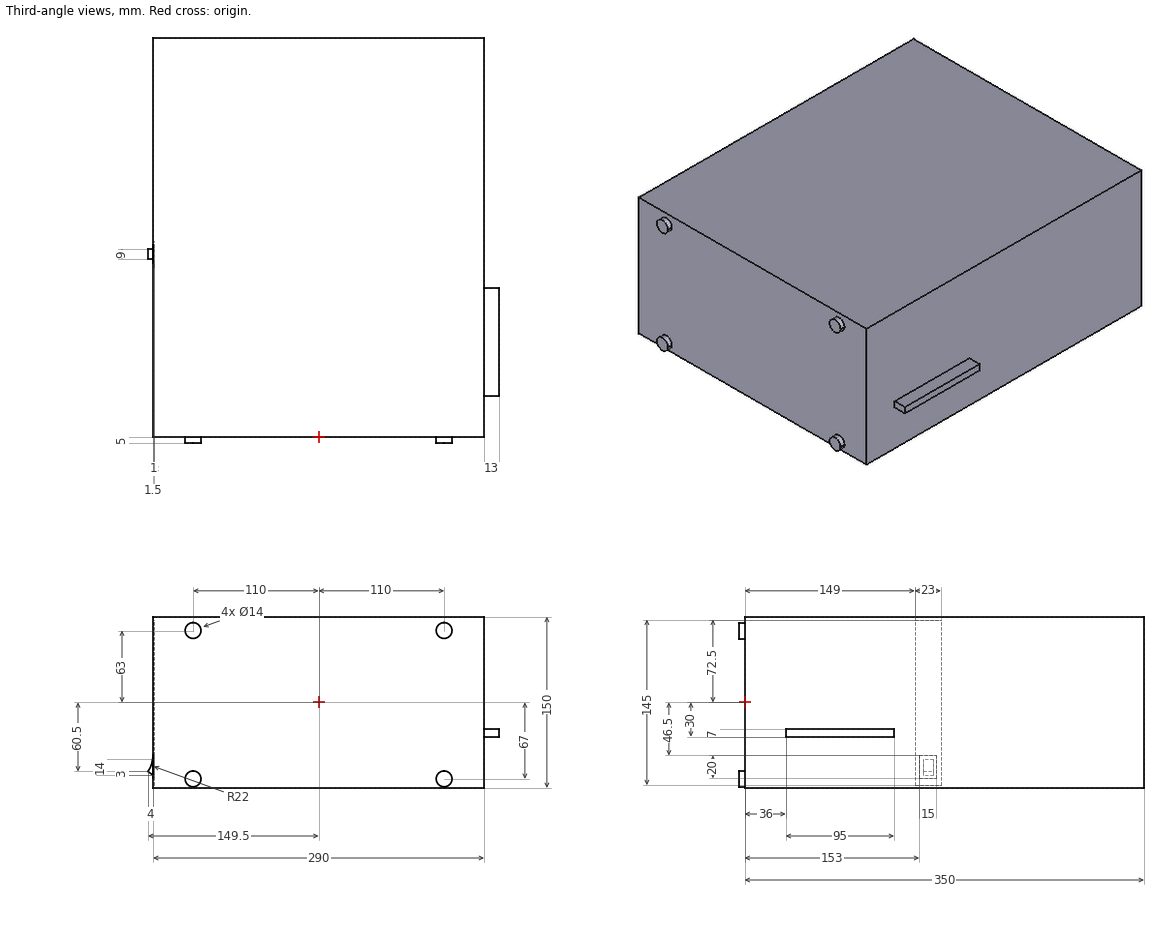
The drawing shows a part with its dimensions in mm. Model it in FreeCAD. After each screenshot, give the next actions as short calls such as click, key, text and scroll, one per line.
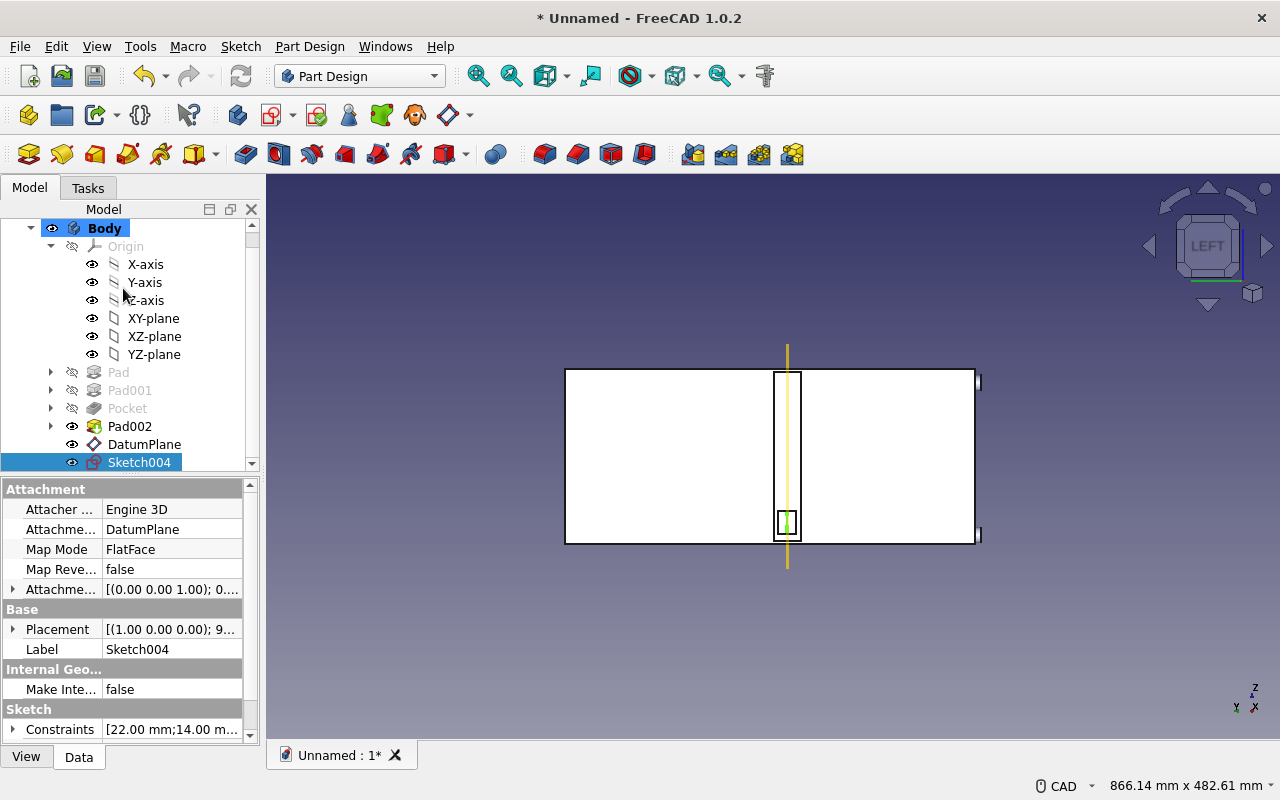
click(29, 154)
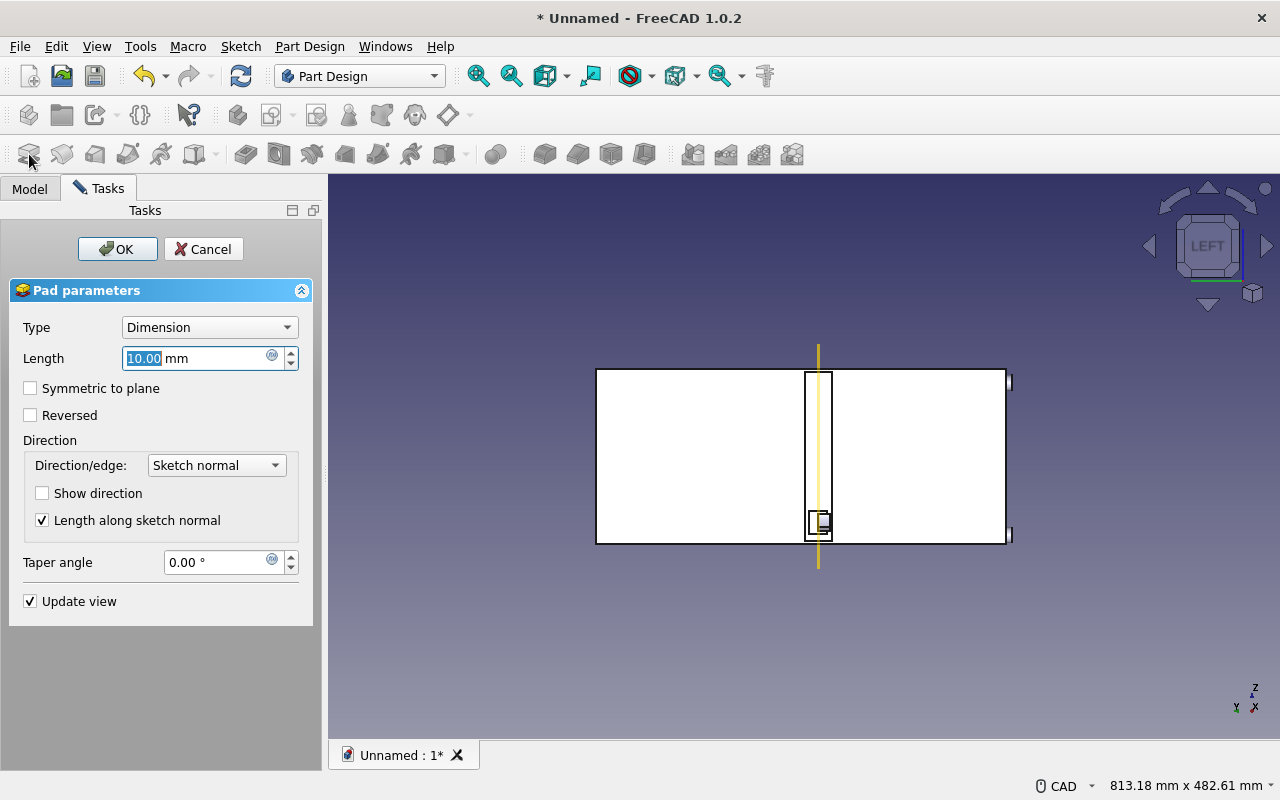
text(9)
key(Tab)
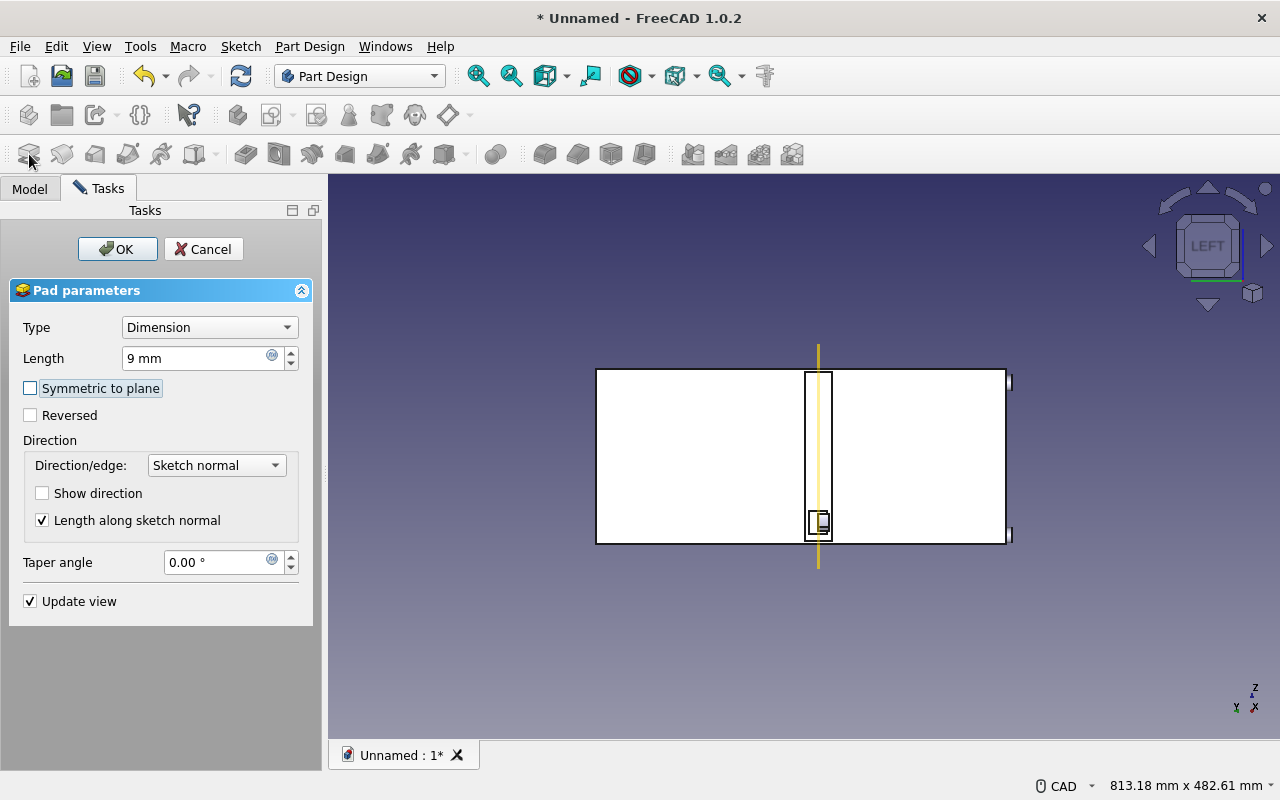
click(31, 388)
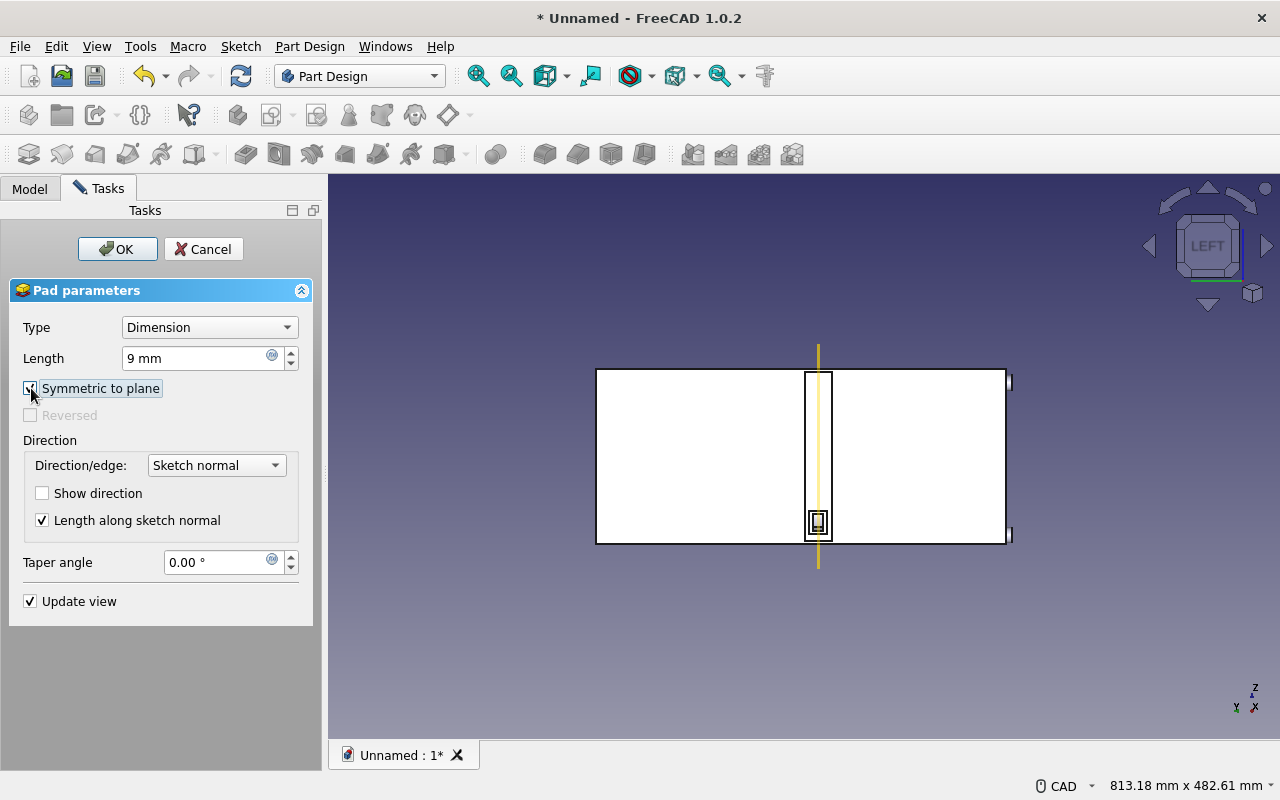
click(118, 249)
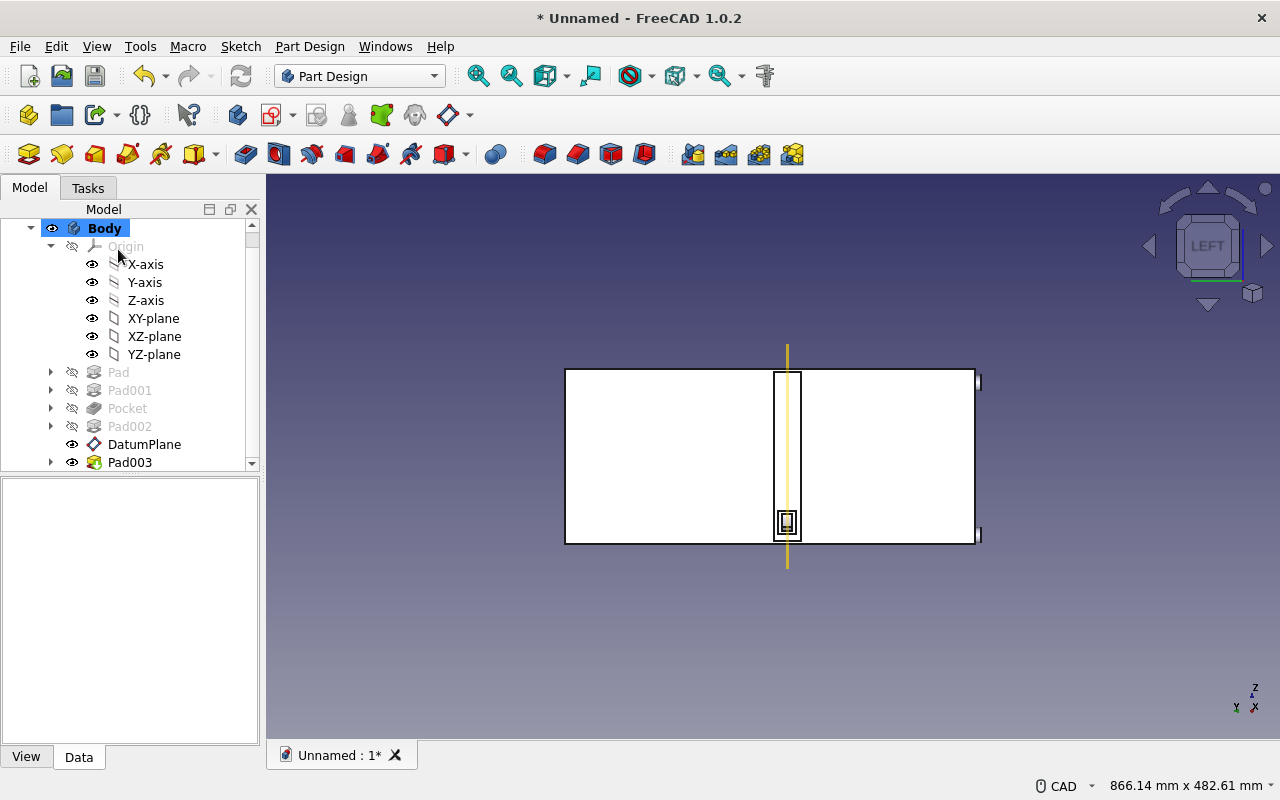
click(117, 444)
key(space)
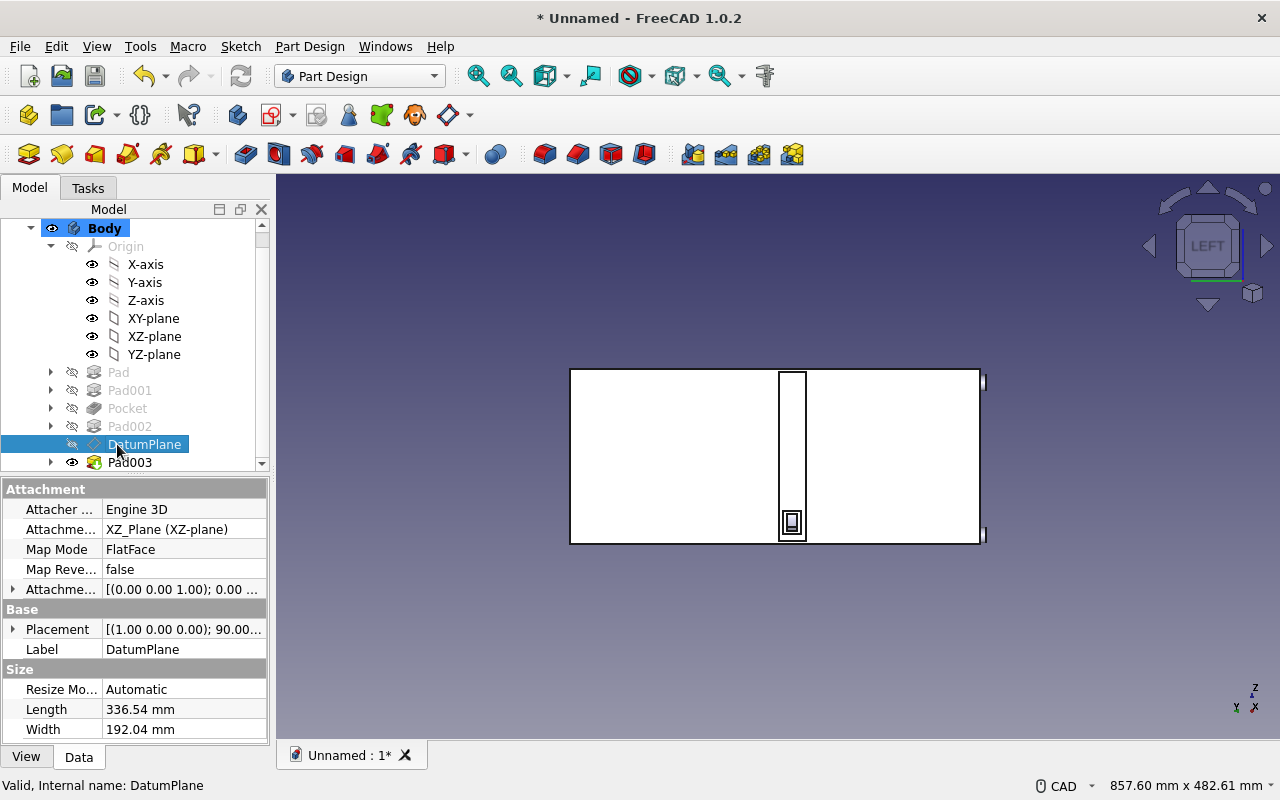
click(479, 76)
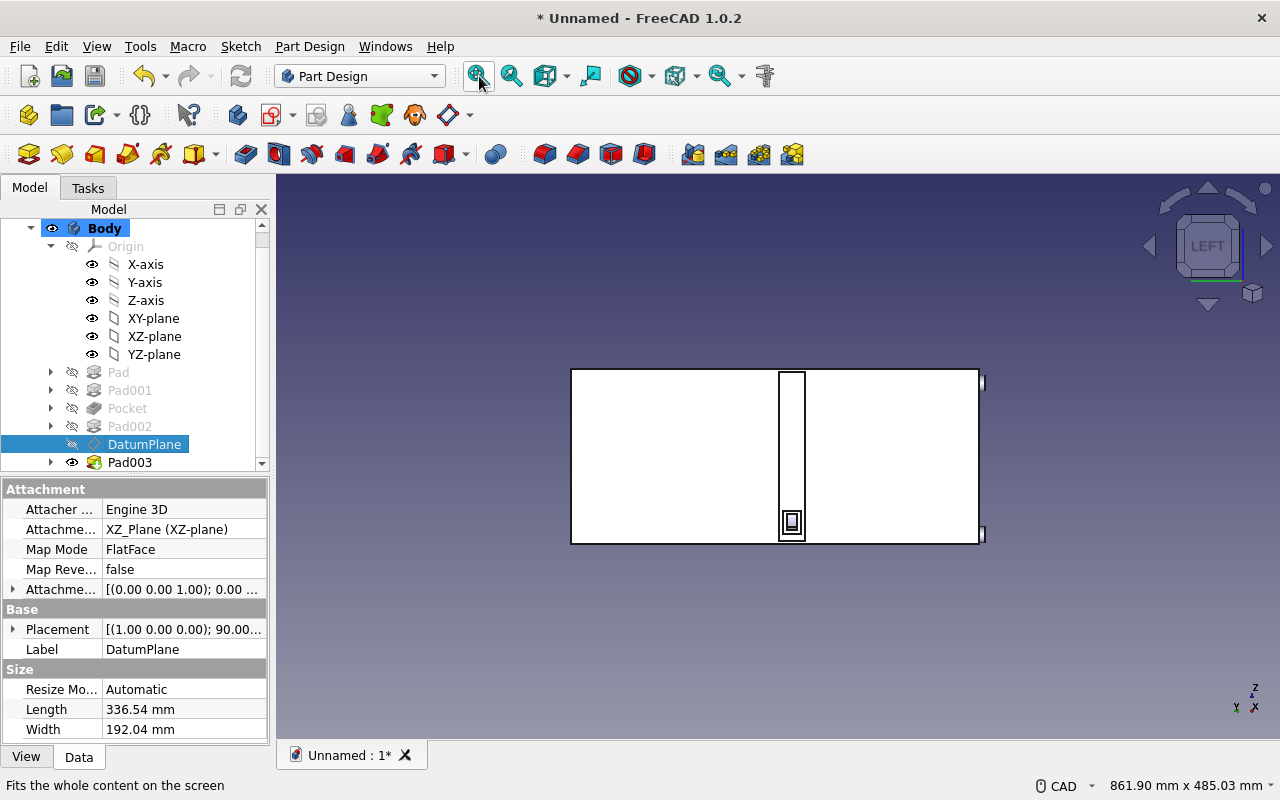
key(0)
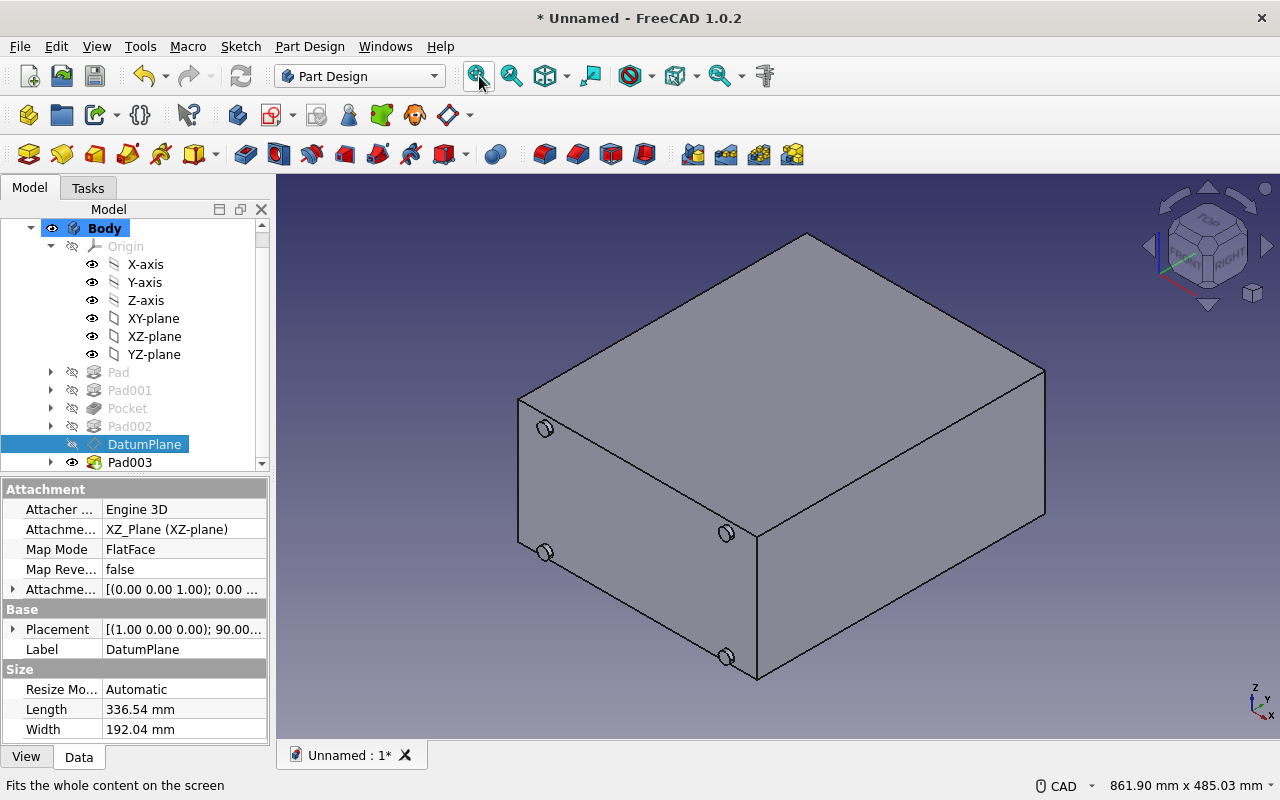
click(860, 548)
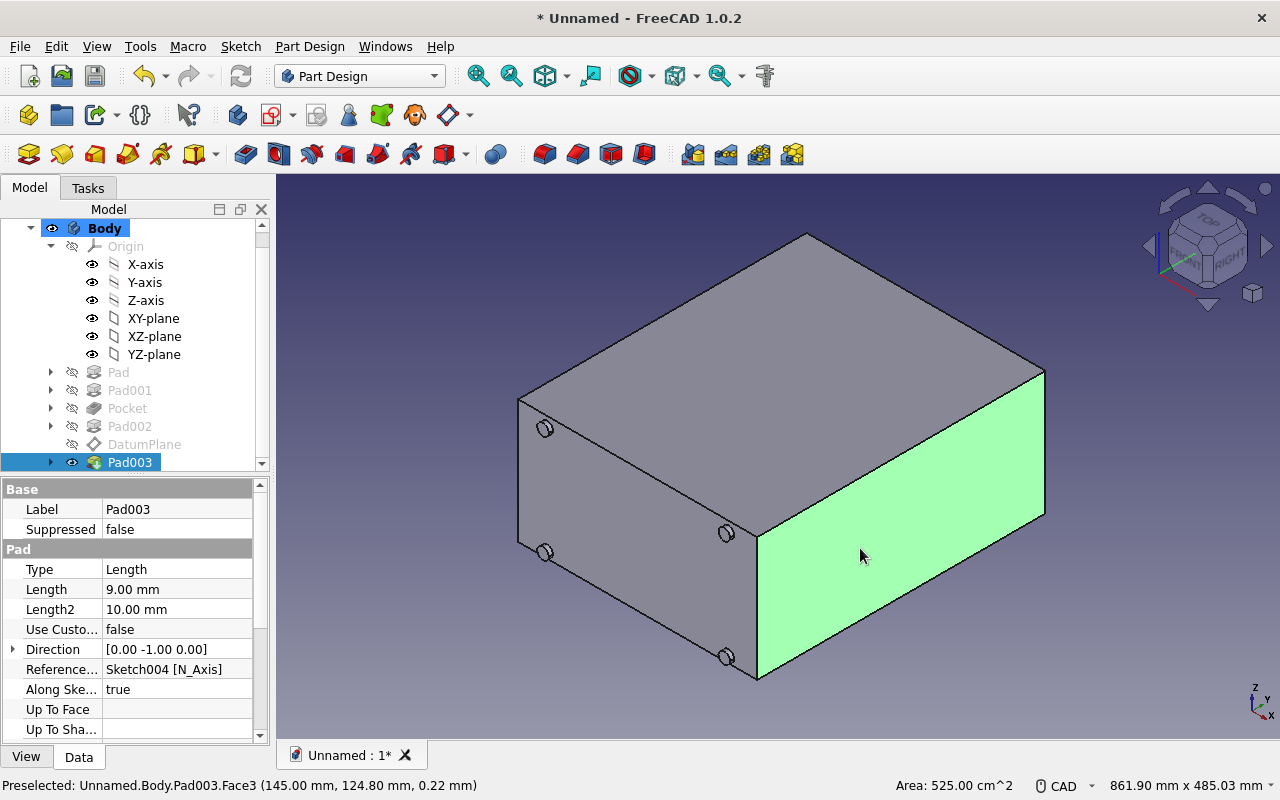
click(270, 116)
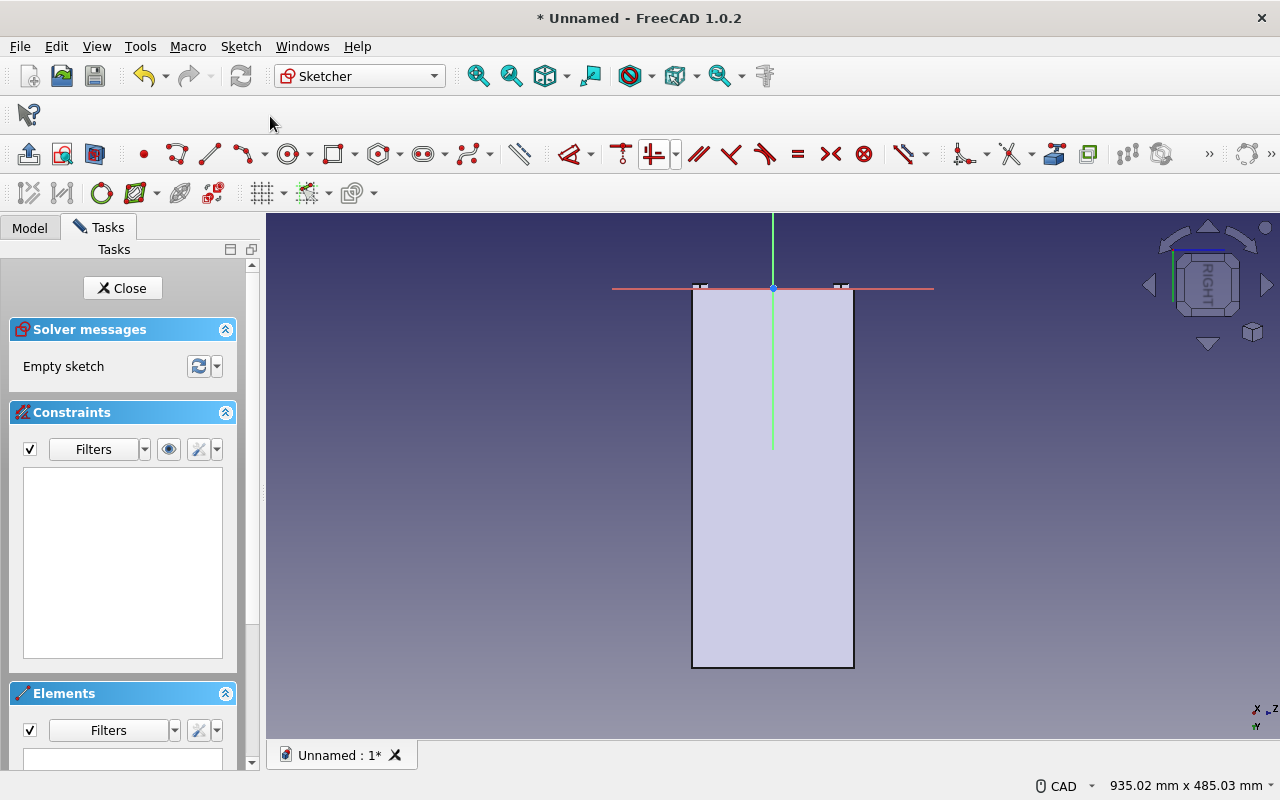
scroll(799, 265, up, 4)